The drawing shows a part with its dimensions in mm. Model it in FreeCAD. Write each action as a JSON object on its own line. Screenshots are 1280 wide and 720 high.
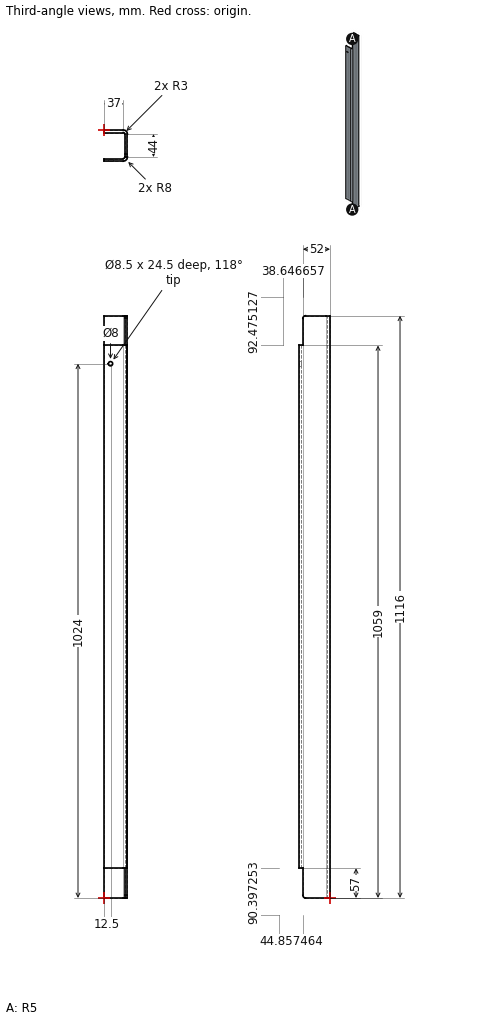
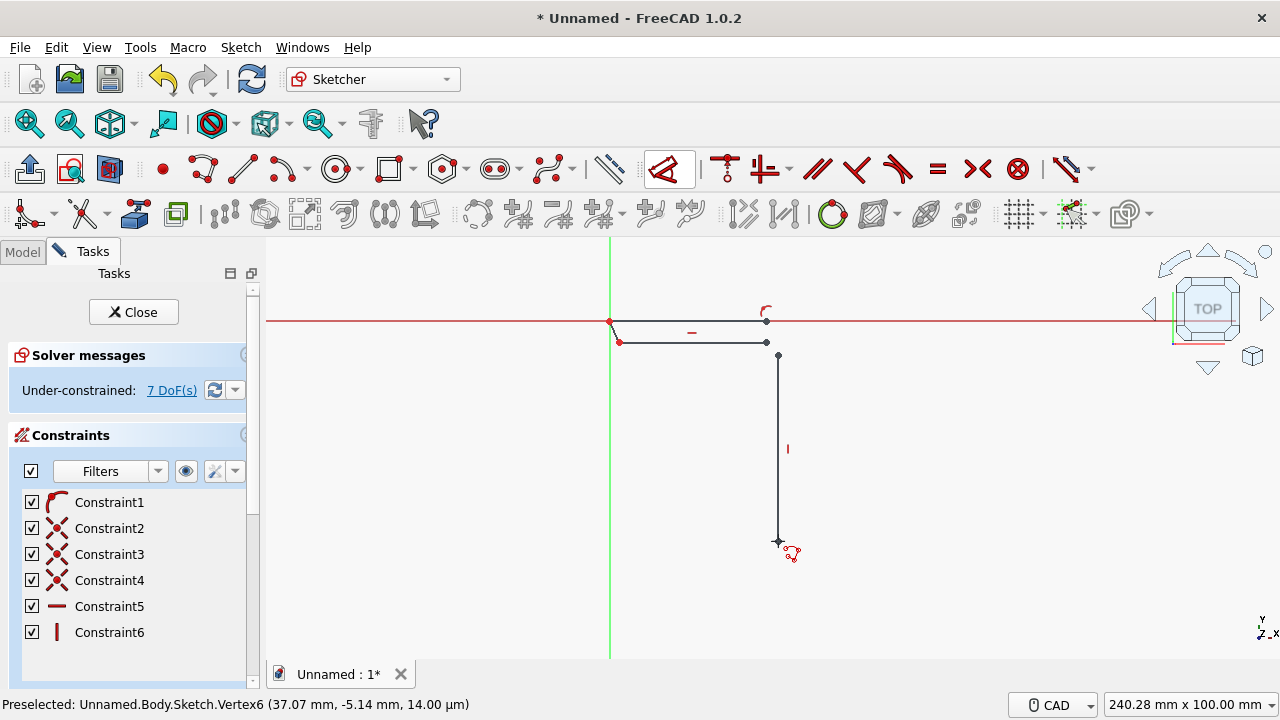
{"action": "left_click", "coordinate": [766, 553]}
{"action": "left_click", "coordinate": [610, 553]}
{"action": "left_click", "coordinate": [619, 575]}
{"action": "left_click", "coordinate": [766, 575]}
{"action": "right_click", "coordinate": [766, 575]}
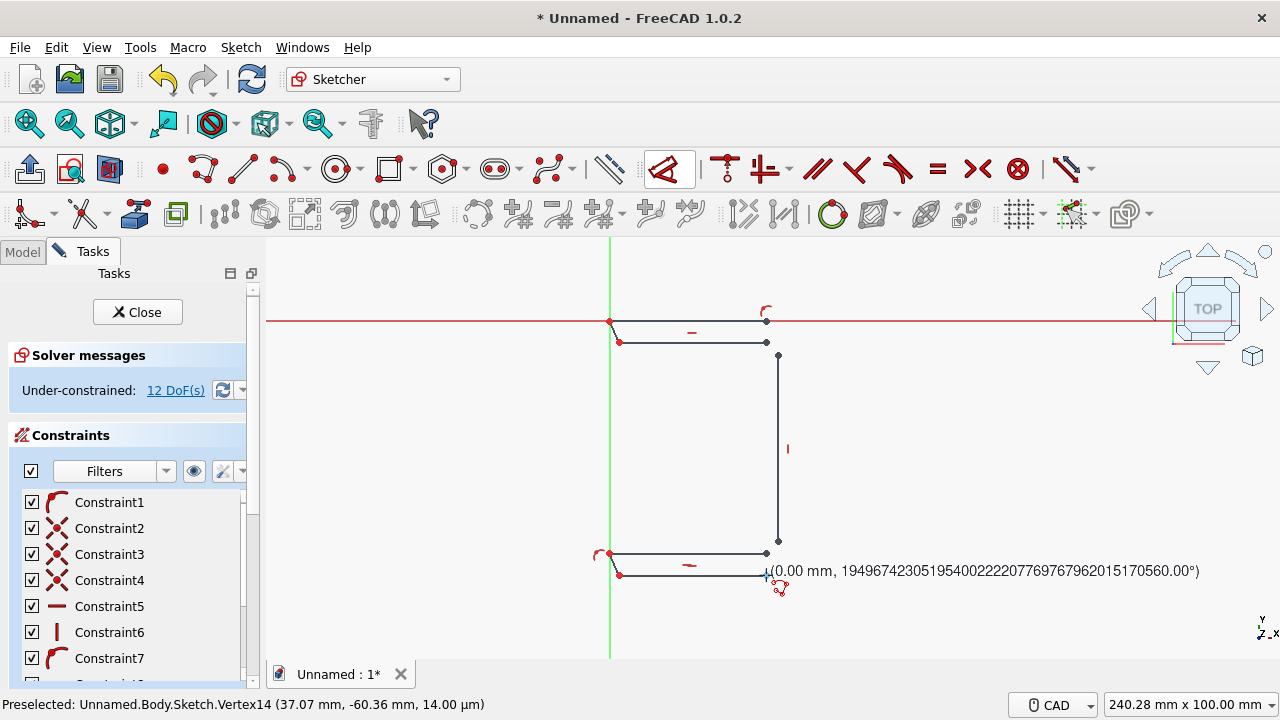
{"action": "key", "text": "g l"}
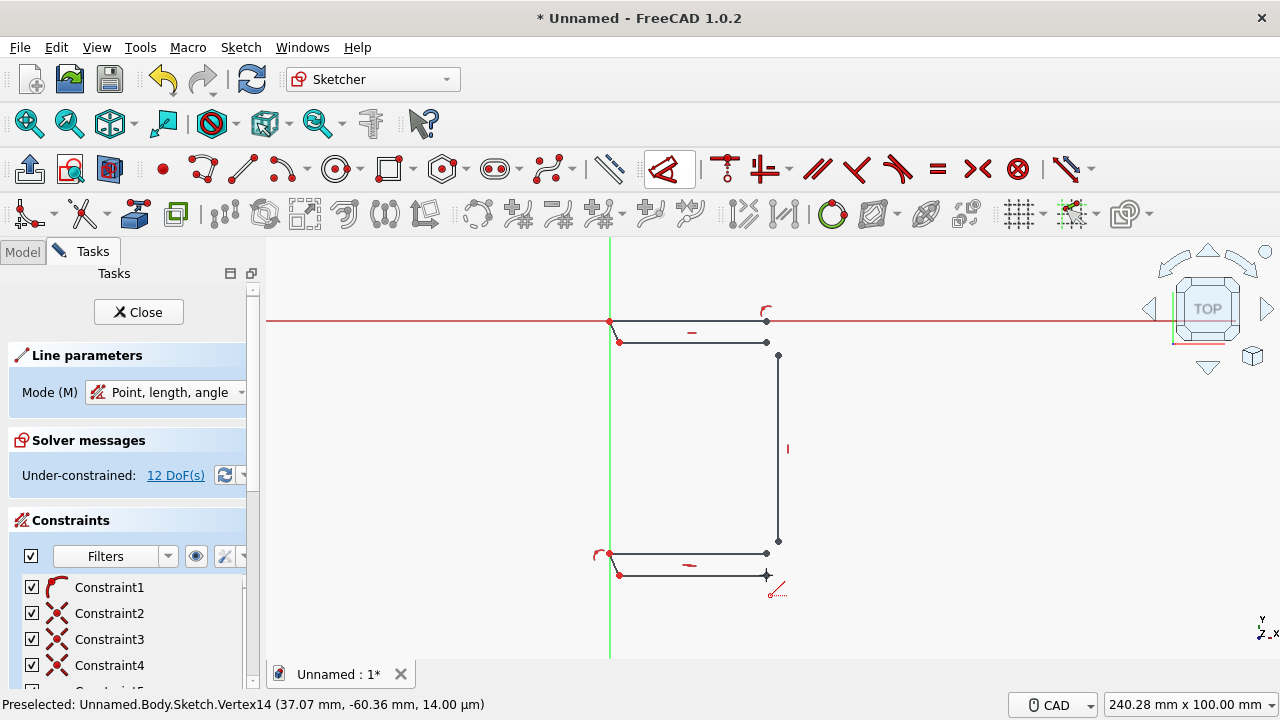
{"action": "left_click", "coordinate": [799, 541]}
{"action": "left_click", "coordinate": [799, 355]}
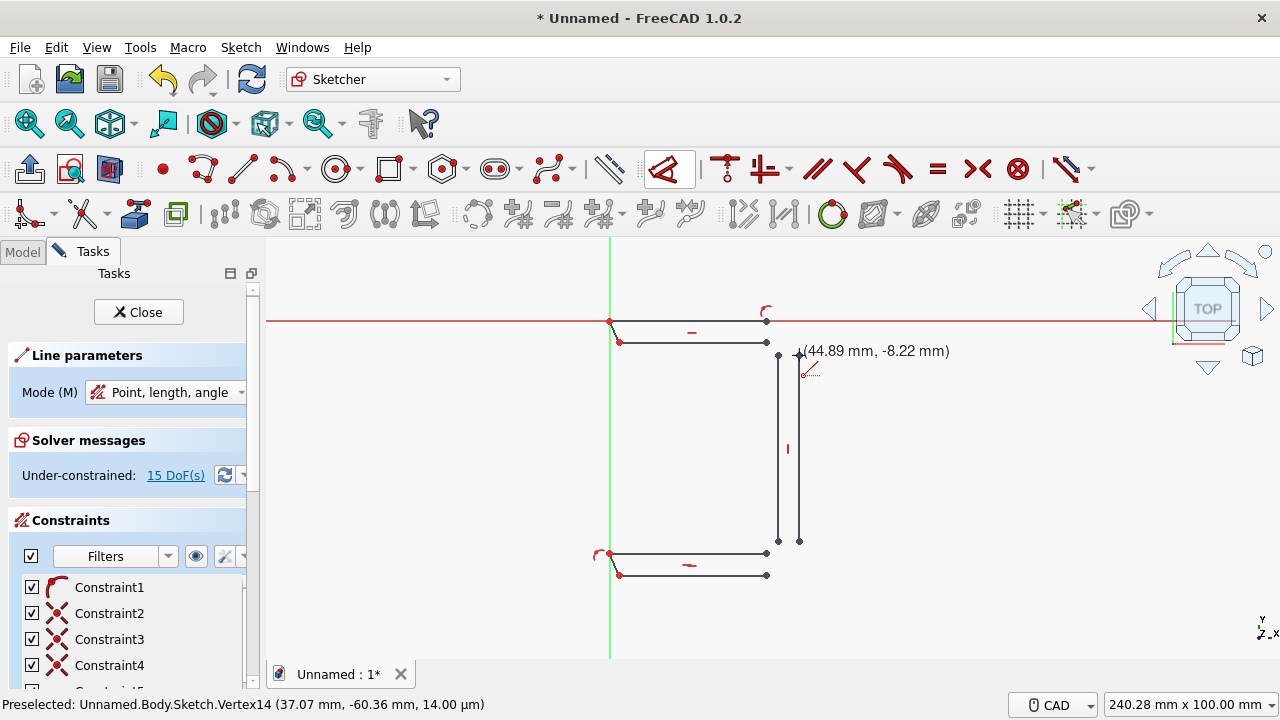
{"action": "left_click", "coordinate": [310, 170]}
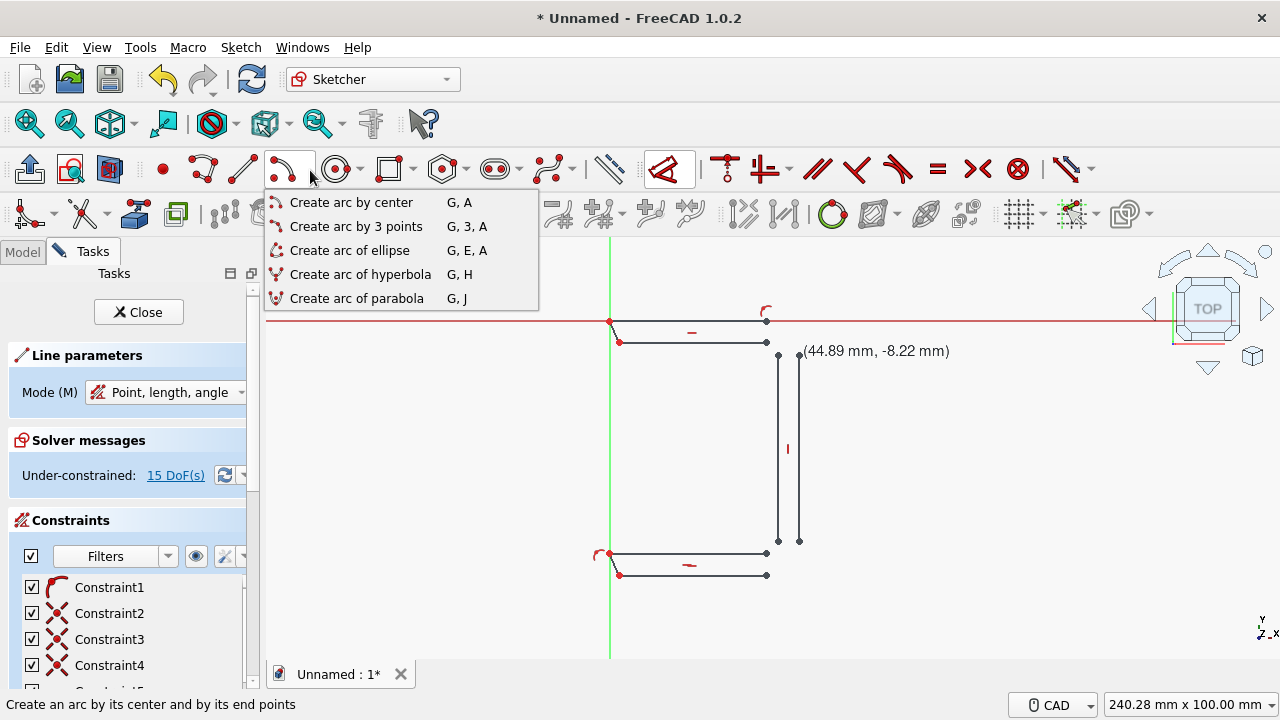
{"action": "left_click", "coordinate": [402, 226]}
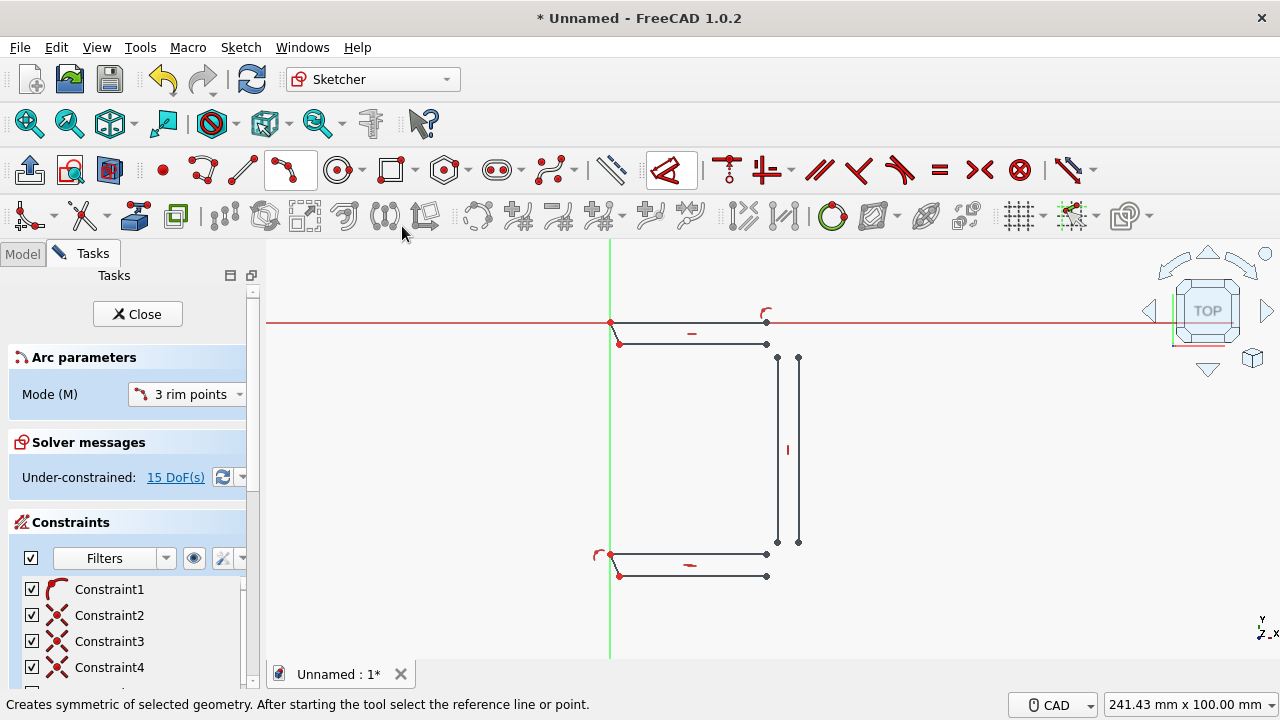
{"action": "left_click", "coordinate": [766, 344]}
{"action": "left_click", "coordinate": [778, 357]}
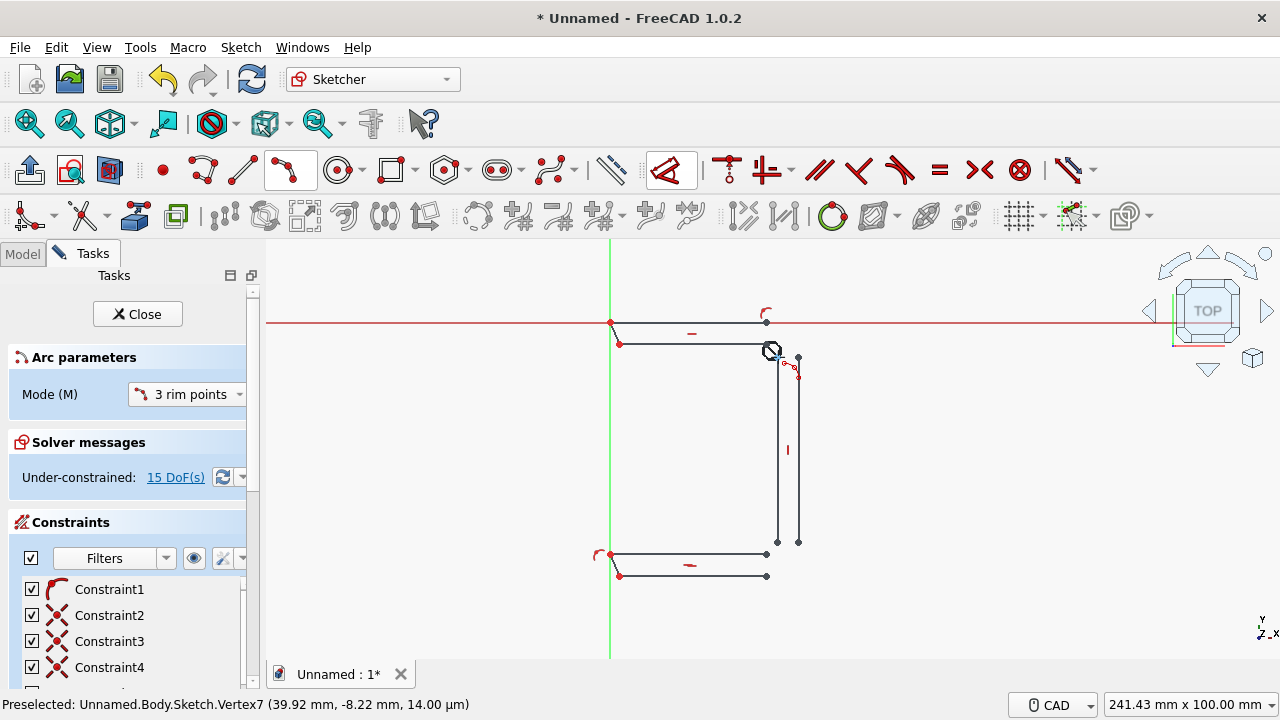
{"action": "scroll", "coordinate": [775, 348], "scroll_direction": "up", "scroll_amount": 8}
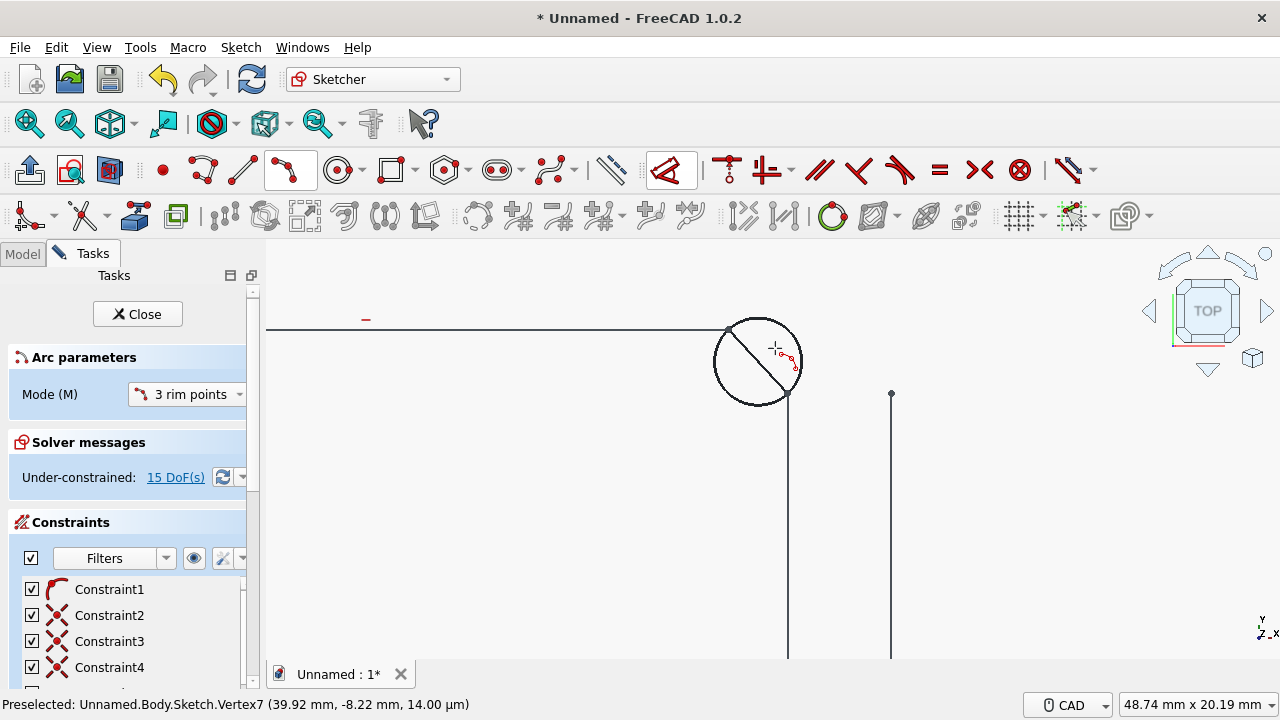
{"action": "left_click", "coordinate": [771, 345]}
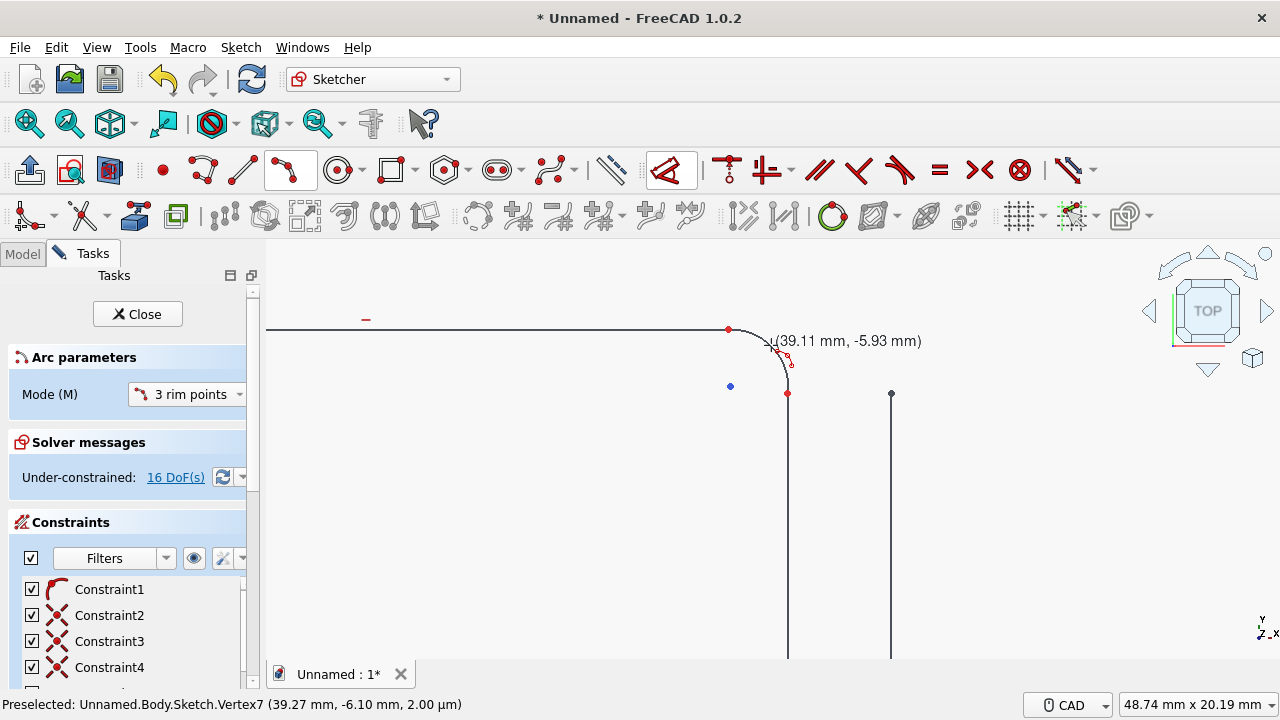
{"action": "scroll", "coordinate": [775, 348], "scroll_direction": "down", "scroll_amount": 8}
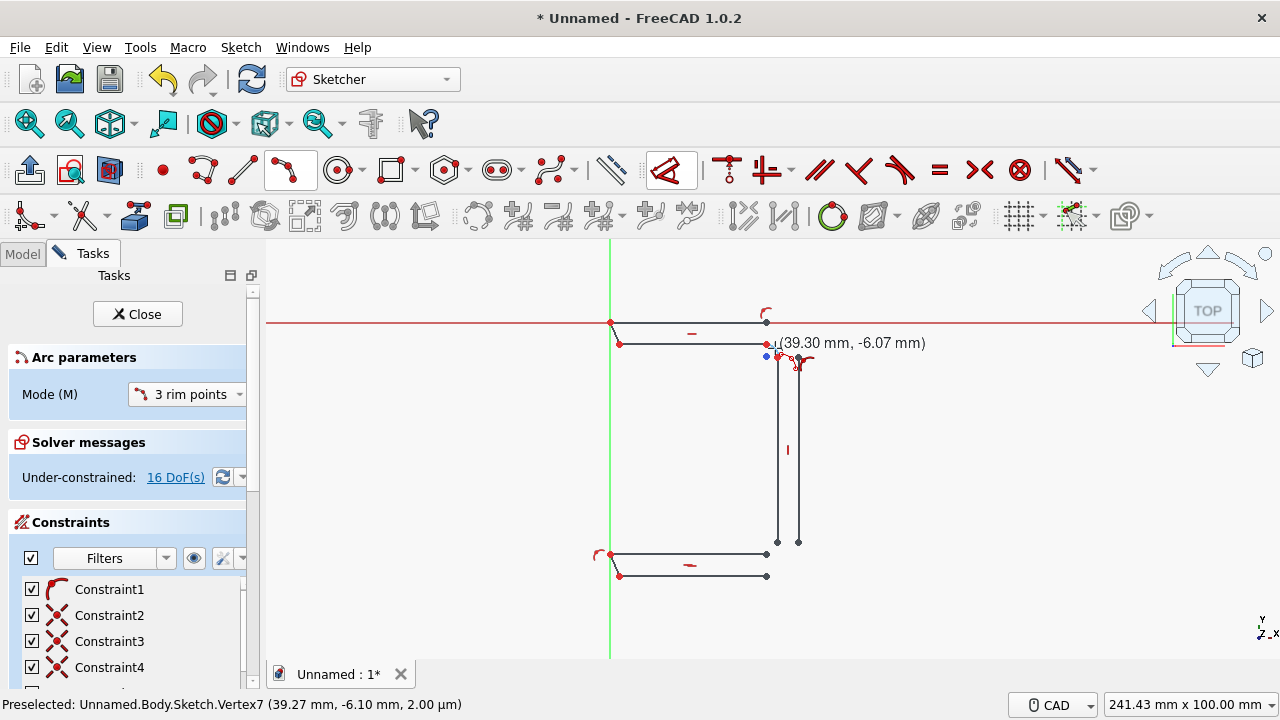
{"action": "left_click", "coordinate": [778, 543]}
{"action": "left_click", "coordinate": [766, 554]}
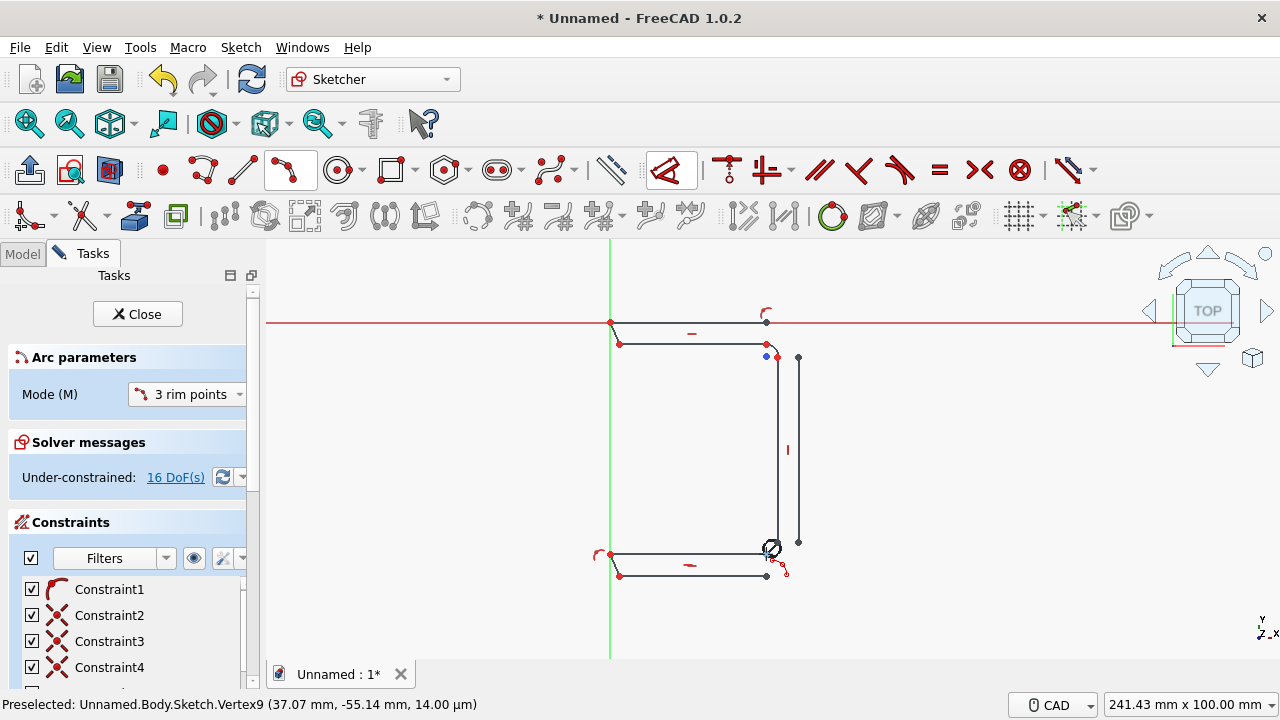
{"action": "scroll", "coordinate": [775, 550], "scroll_direction": "up", "scroll_amount": 8}